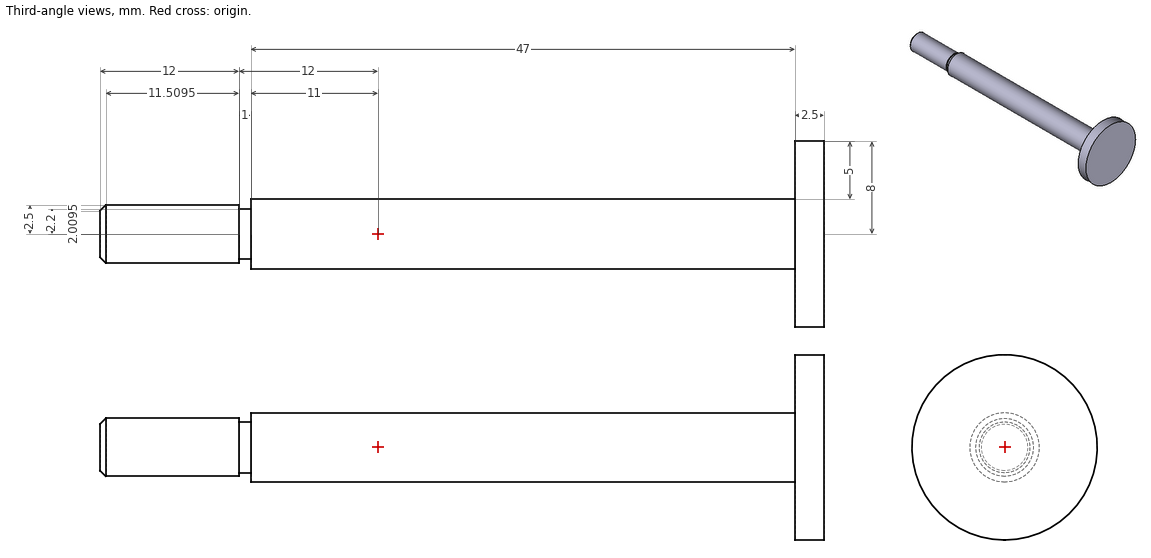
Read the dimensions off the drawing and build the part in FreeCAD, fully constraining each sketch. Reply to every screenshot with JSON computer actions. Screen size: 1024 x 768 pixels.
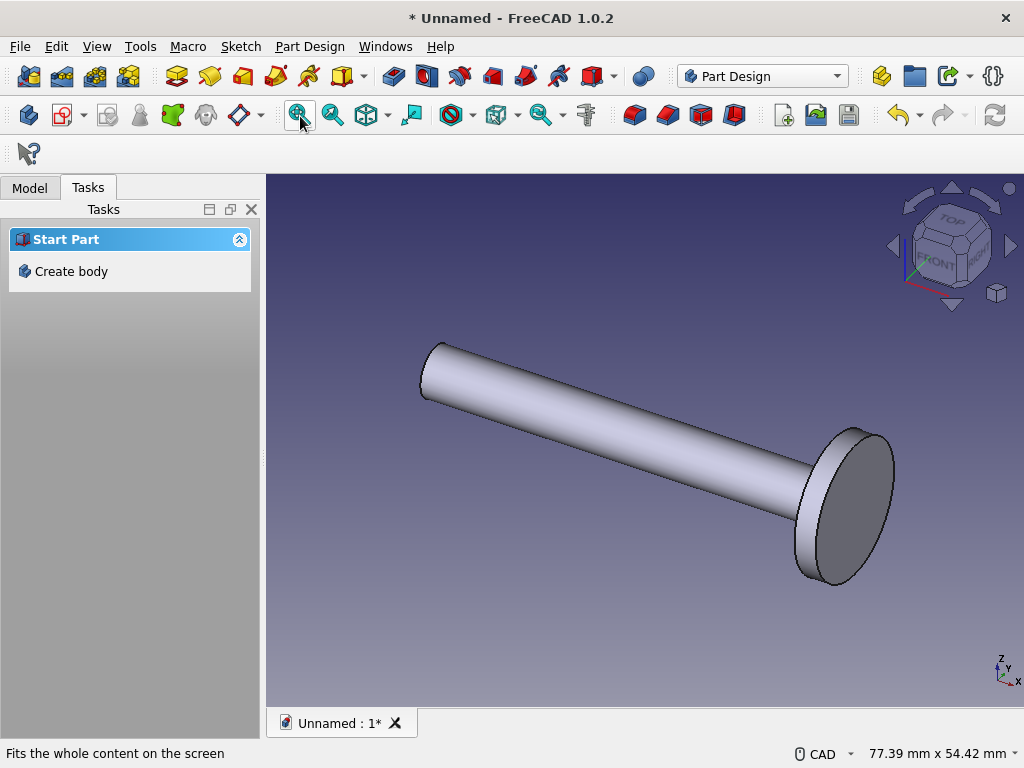
{"action": "left_click", "coordinate": [62, 116]}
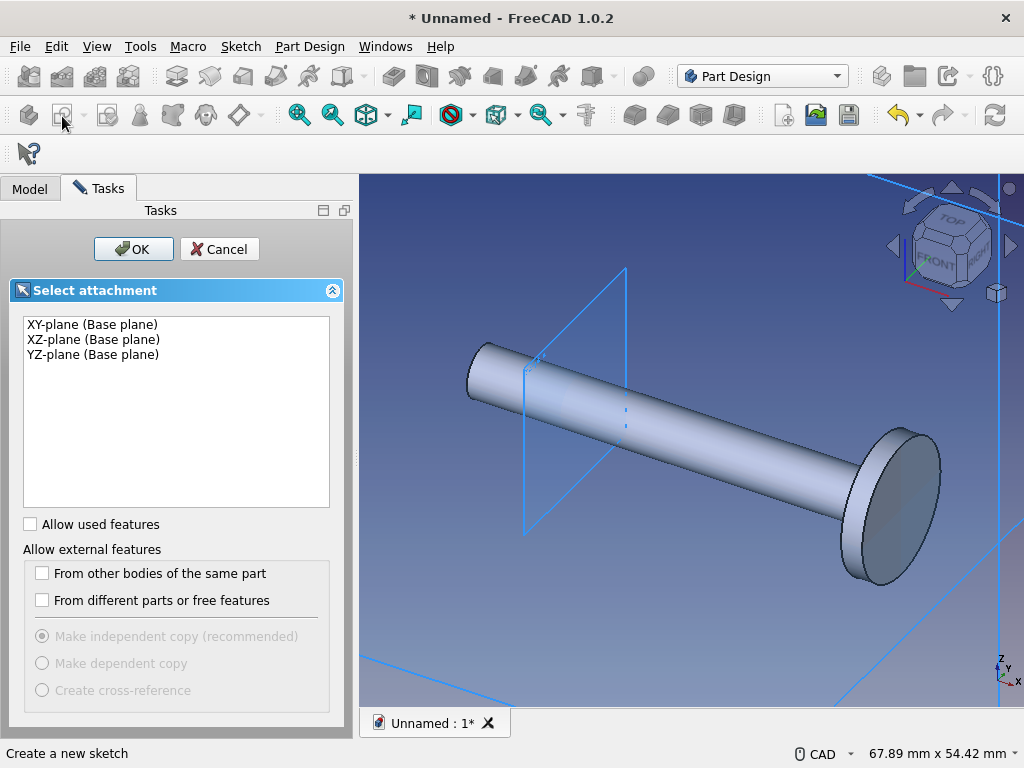
{"action": "left_click", "coordinate": [84, 324]}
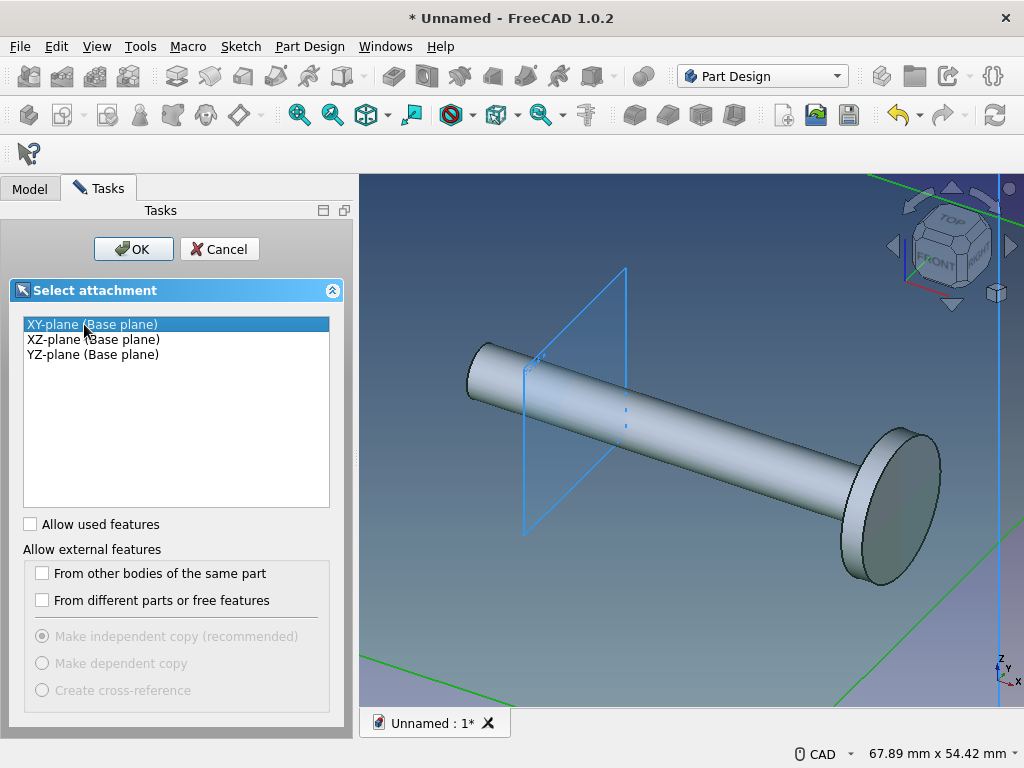
{"action": "left_click", "coordinate": [134, 249]}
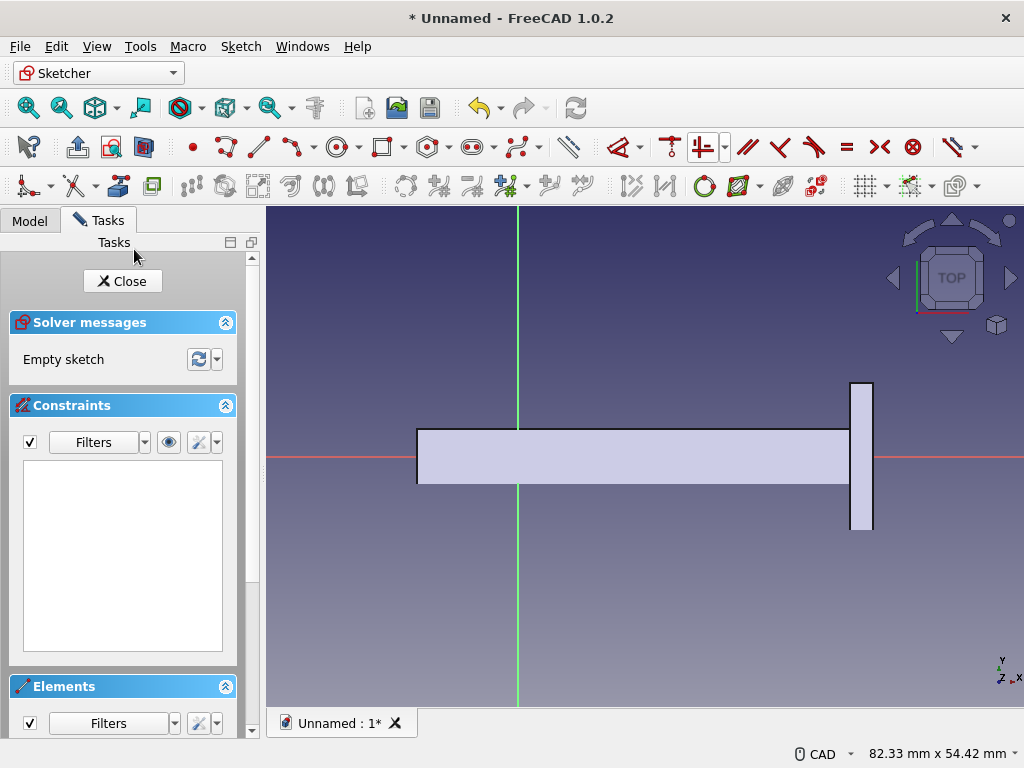
{"action": "left_click", "coordinate": [144, 148]}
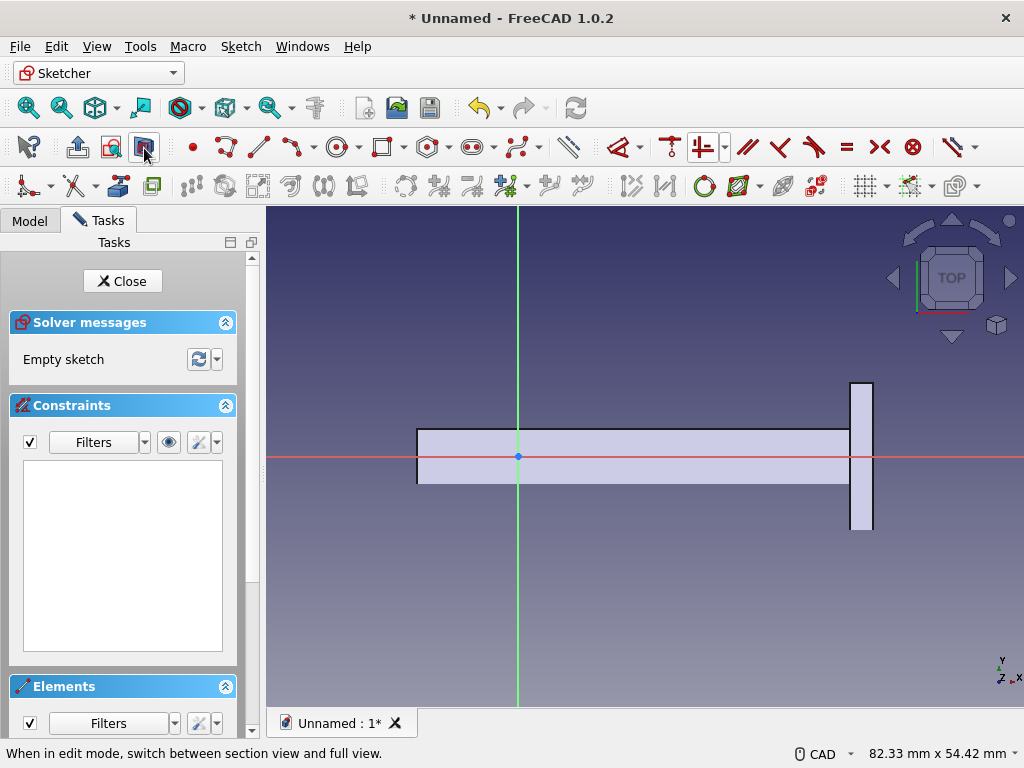
{"action": "scroll", "coordinate": [402, 446], "scroll_direction": "up", "scroll_amount": 14}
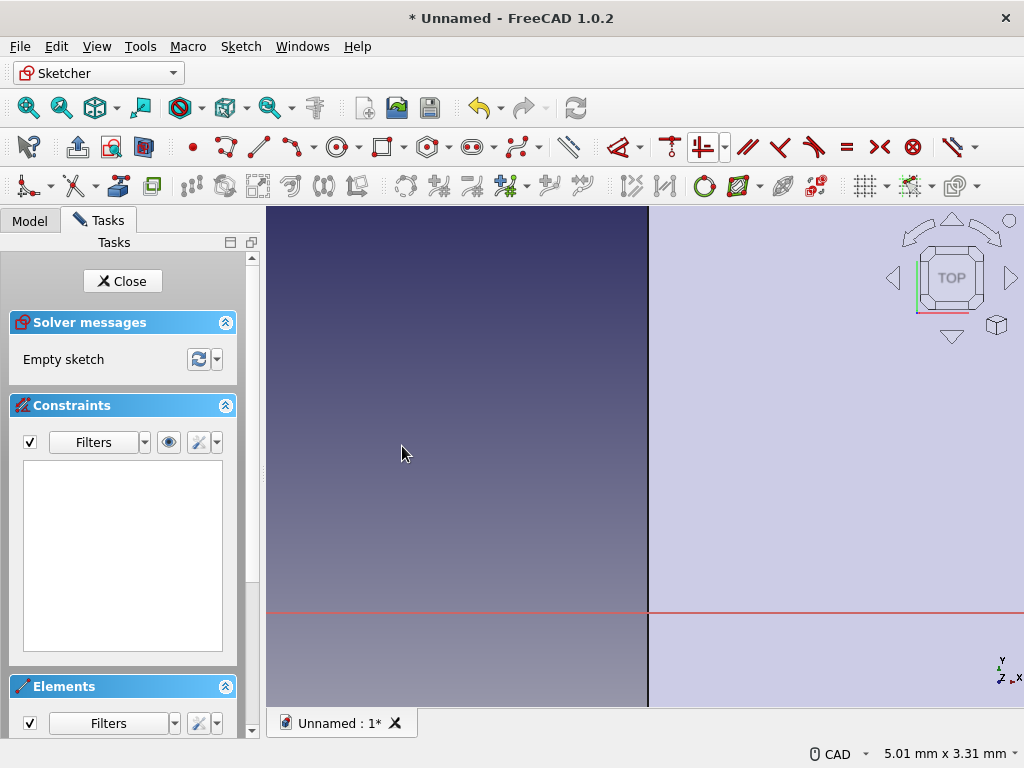
{"action": "key", "text": "g r"}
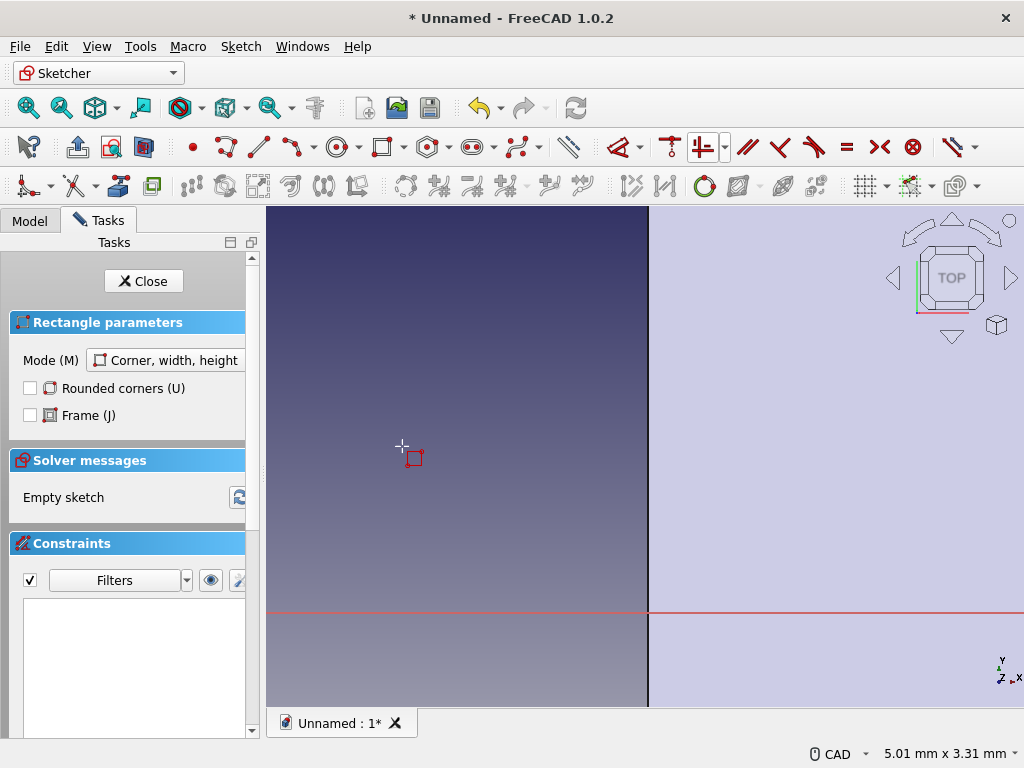
{"action": "left_click", "coordinate": [497, 280]}
{"action": "left_click", "coordinate": [648, 613]}
{"action": "key", "text": "Escape"}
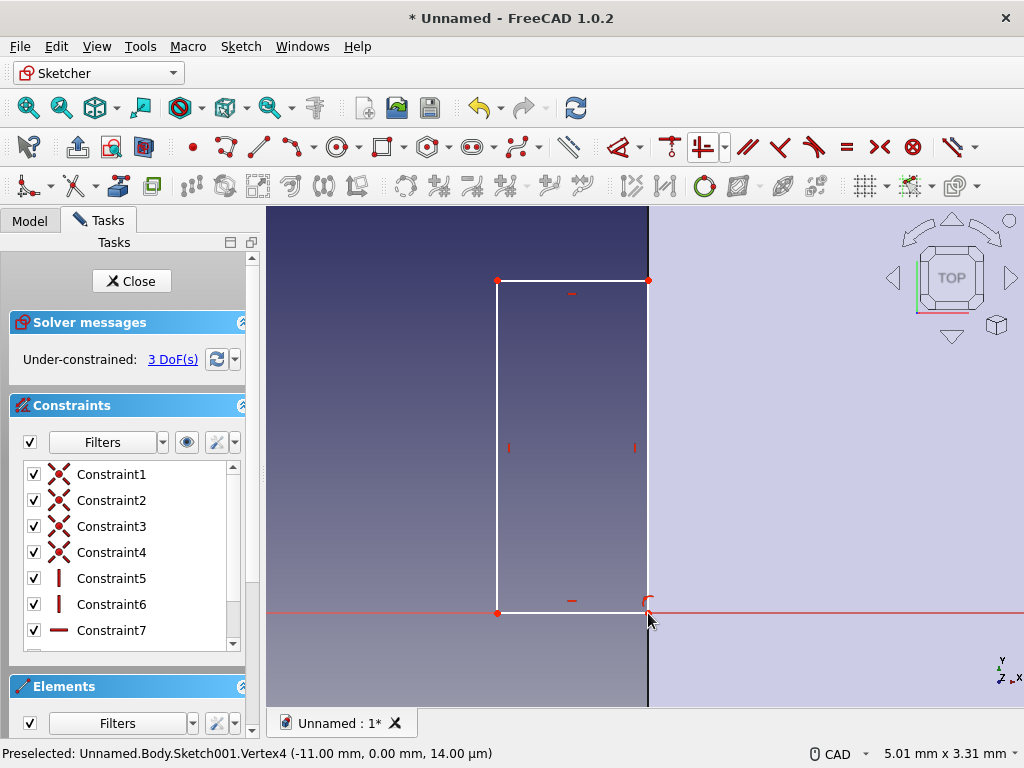
{"action": "key", "text": "d"}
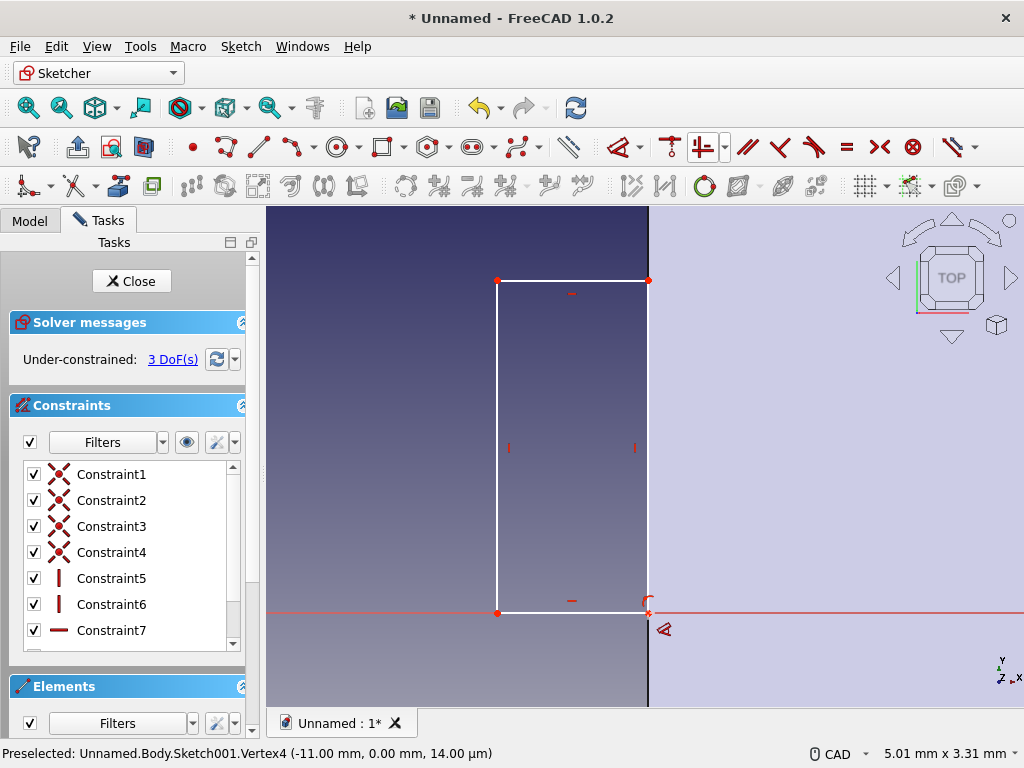
{"action": "left_click", "coordinate": [542, 613]}
{"action": "left_click", "coordinate": [572, 647]}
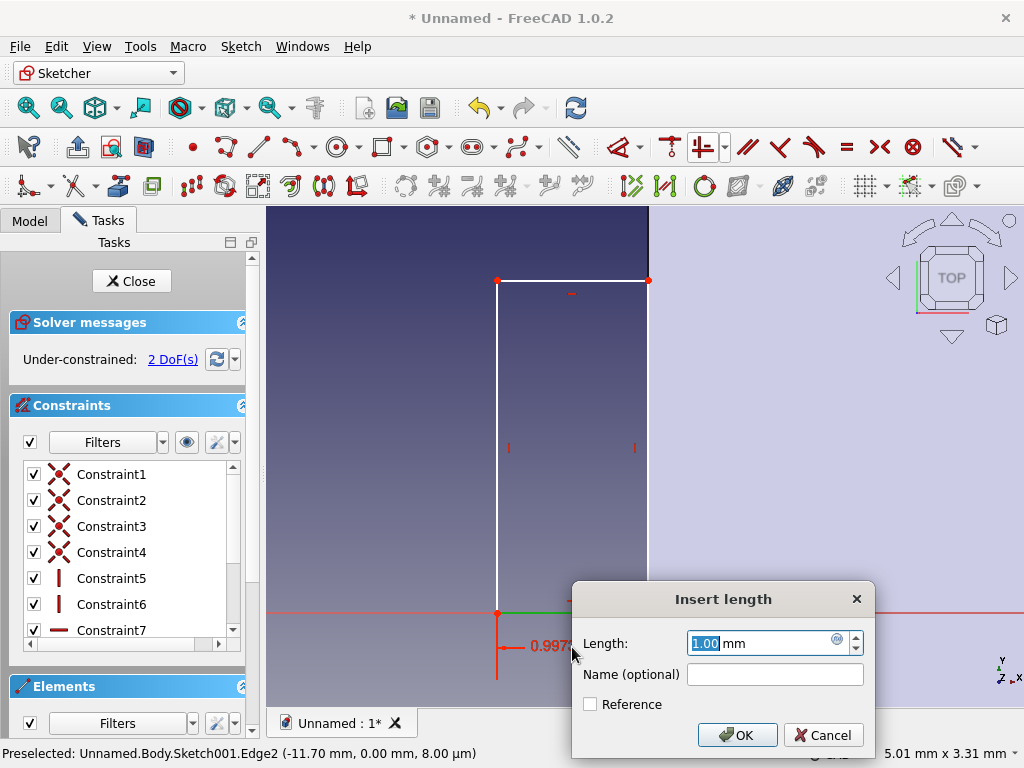
{"action": "type", "text": "1"}
{"action": "key", "text": "Return"}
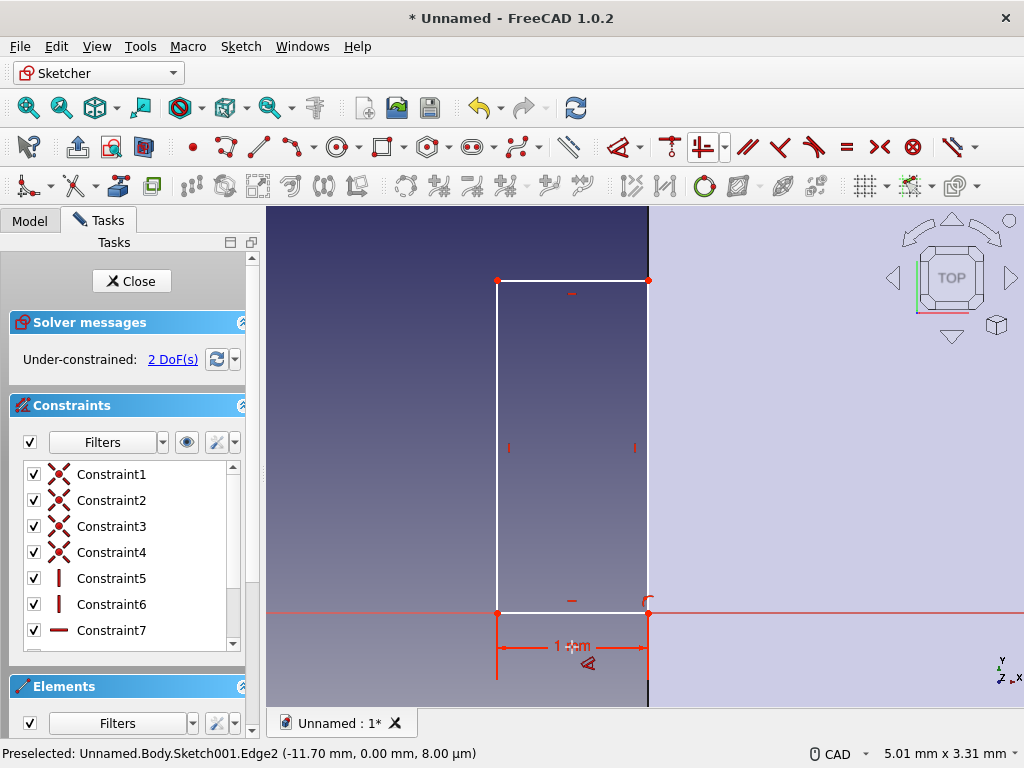
{"action": "left_click", "coordinate": [497, 381]}
{"action": "left_click", "coordinate": [463, 447]}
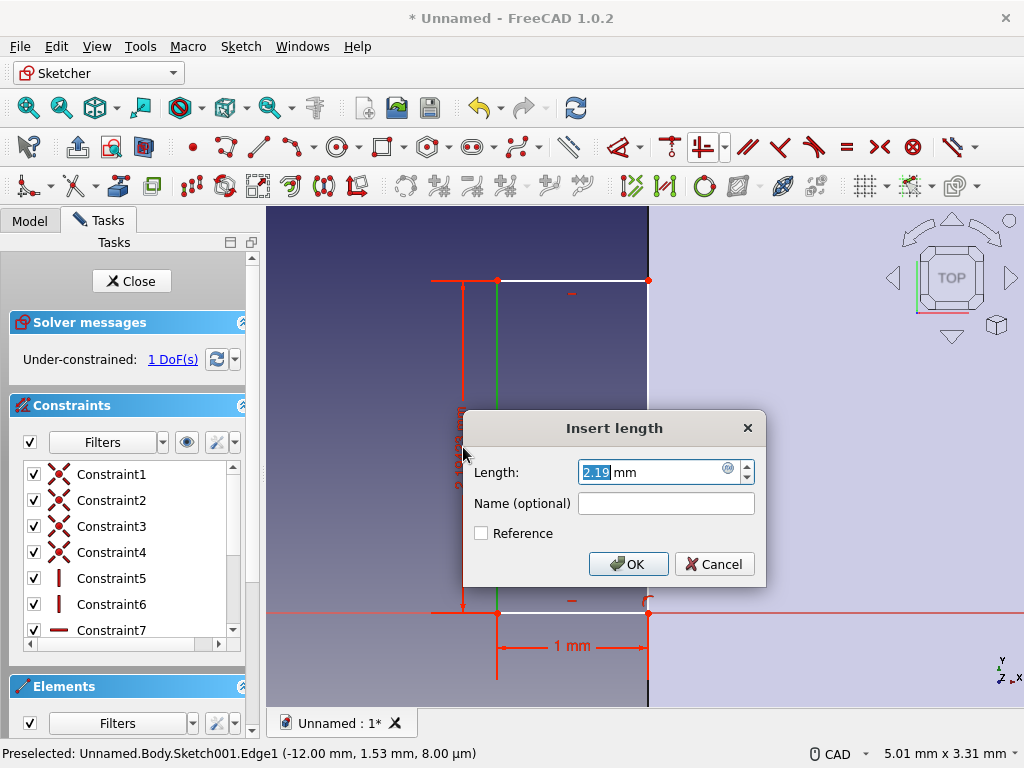
{"action": "type", "text": "2.2"}
{"action": "key", "text": "Return"}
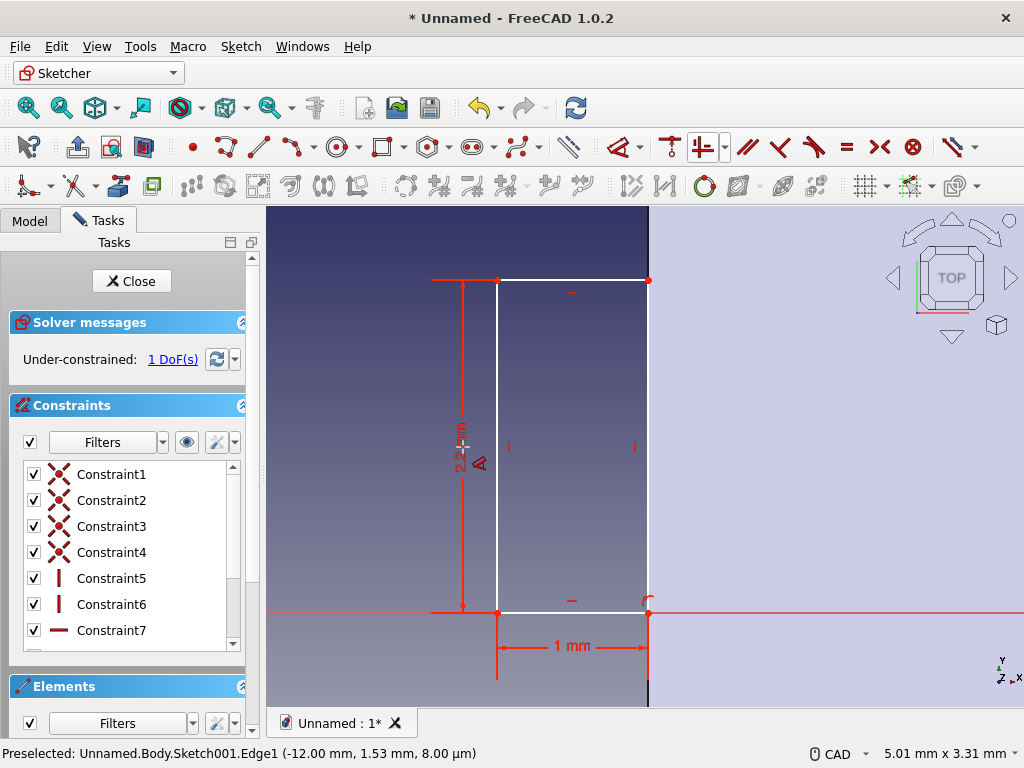
{"action": "left_click", "coordinate": [497, 280]}
{"action": "left_click", "coordinate": [678, 647]}